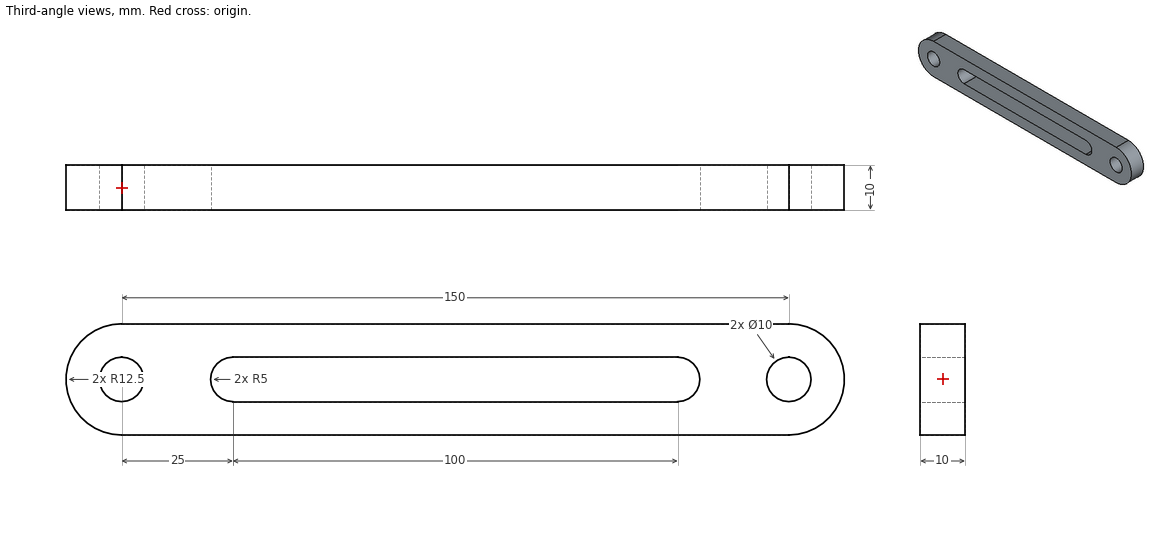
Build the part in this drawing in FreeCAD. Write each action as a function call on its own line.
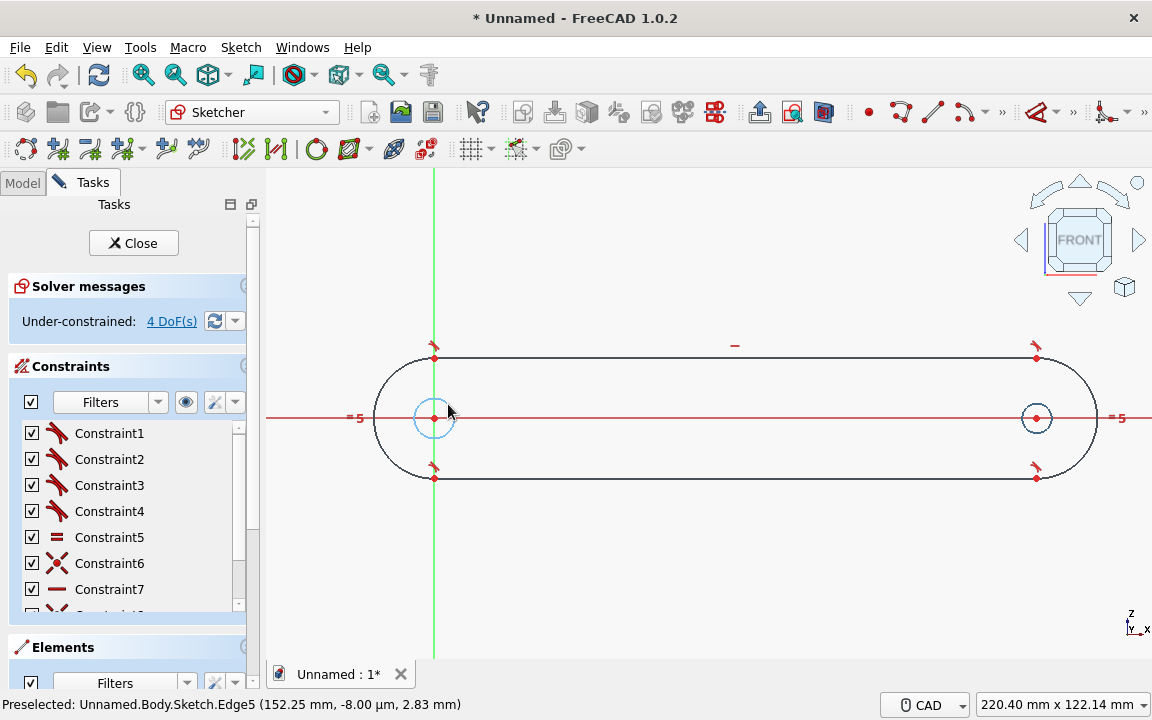
click(448, 404)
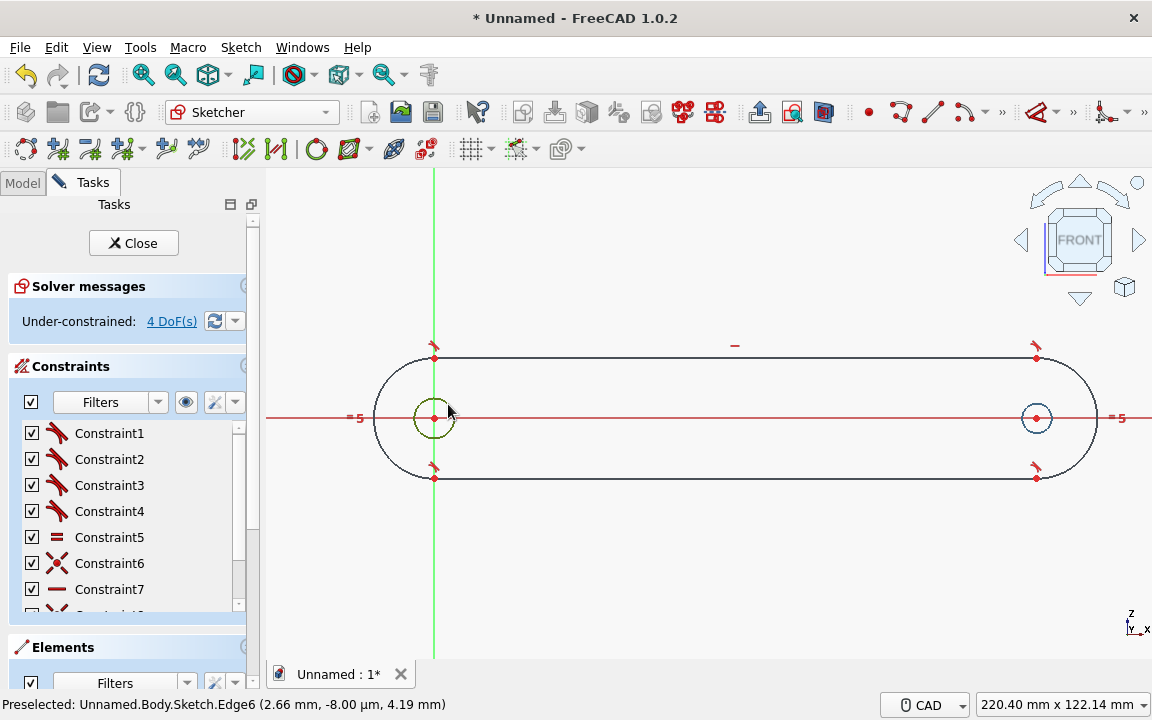
key(e)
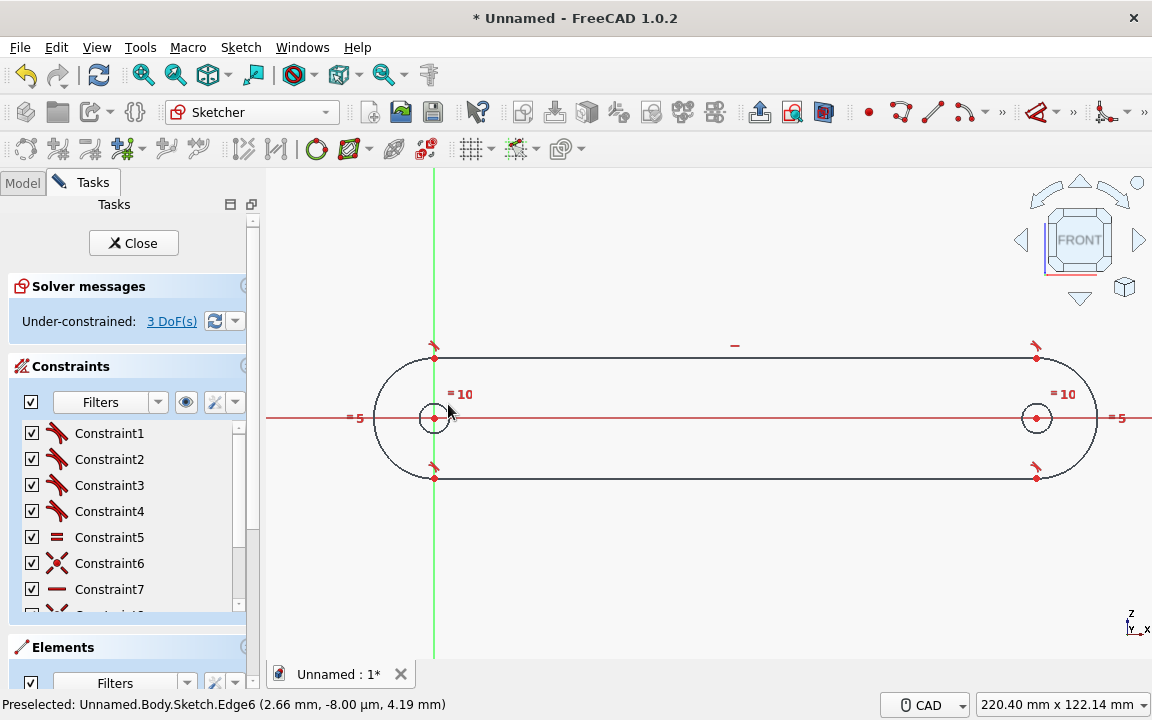
click(1036, 112)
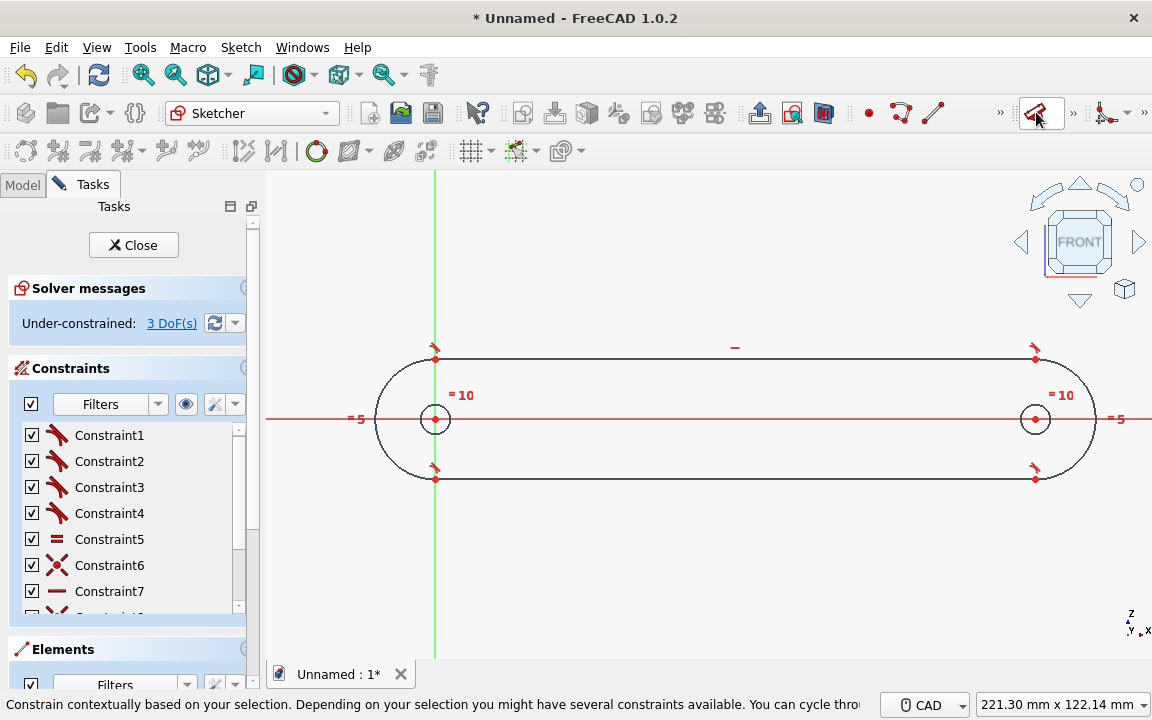
click(387, 384)
click(361, 365)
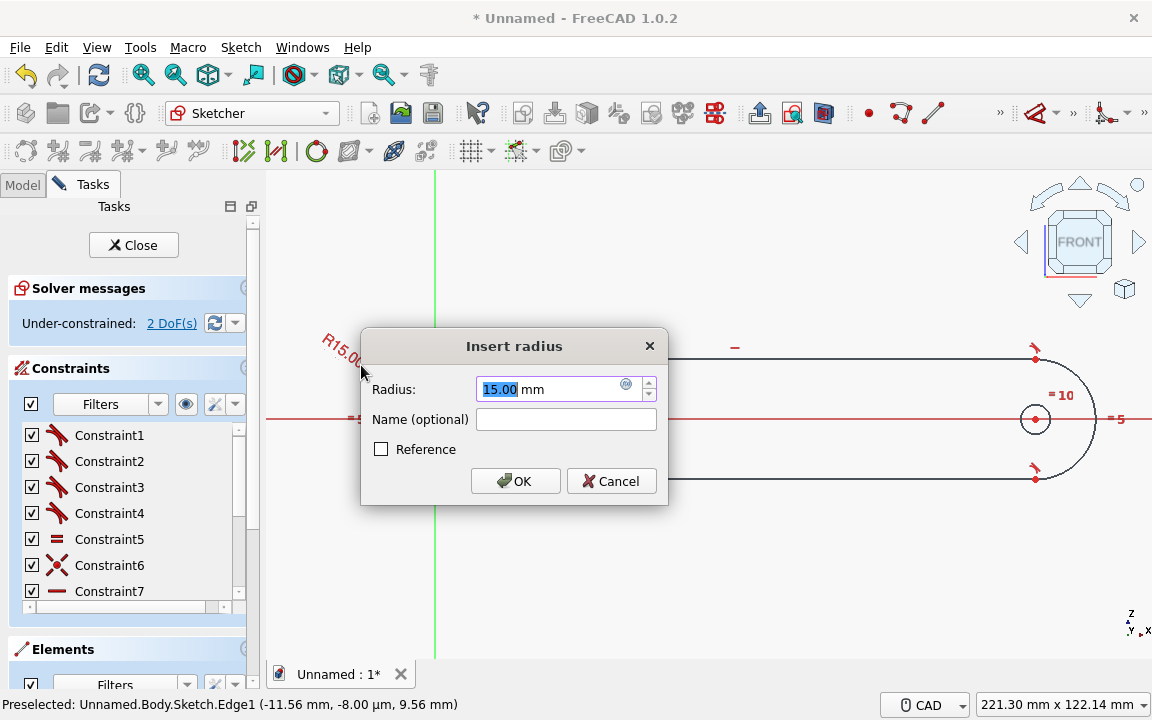
text(12.5)
key(Return)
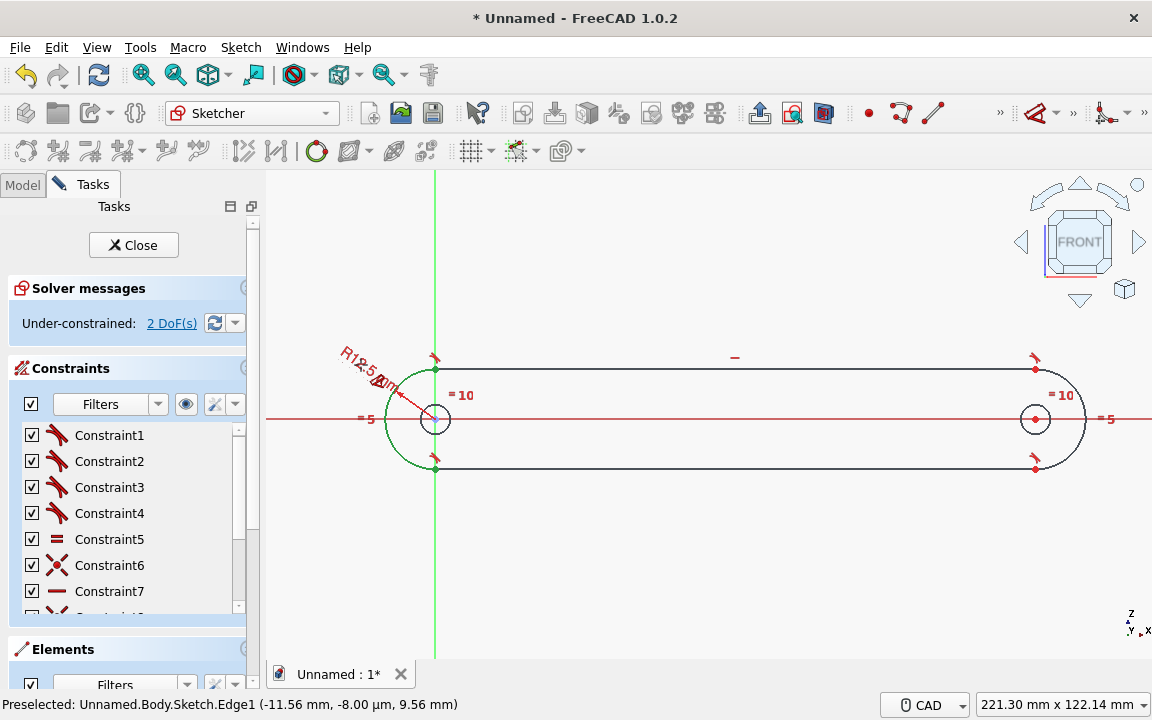
scroll(447, 405, down, 2)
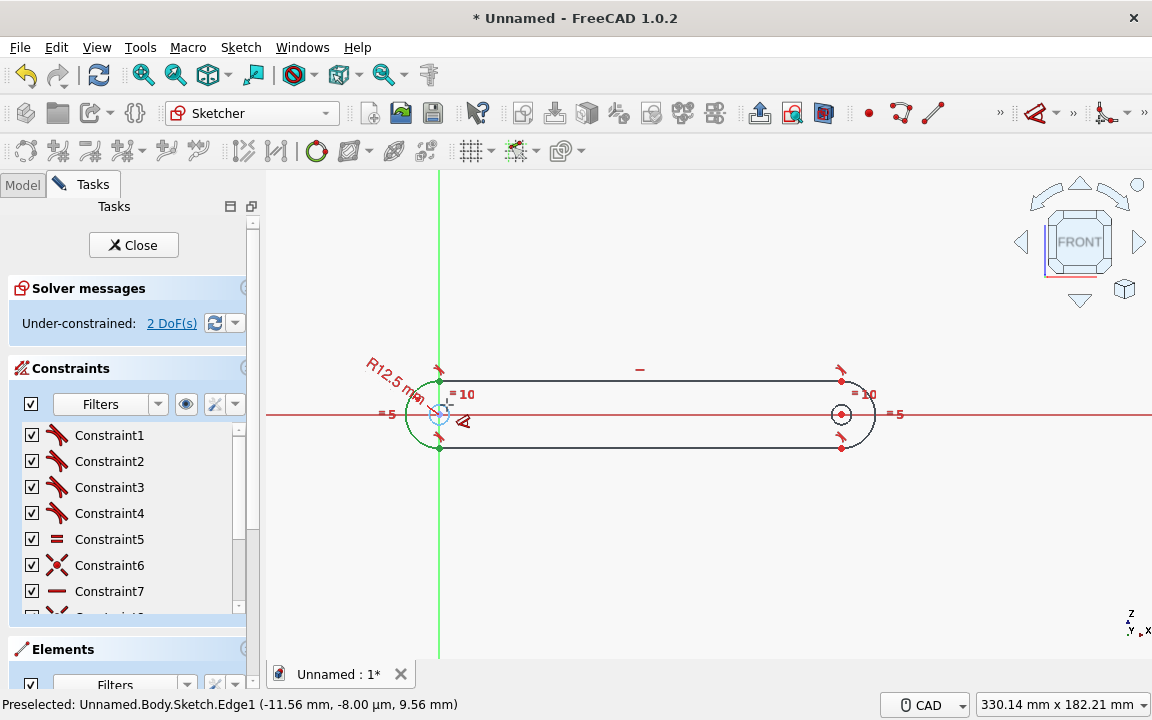
scroll(849, 408, up, 4)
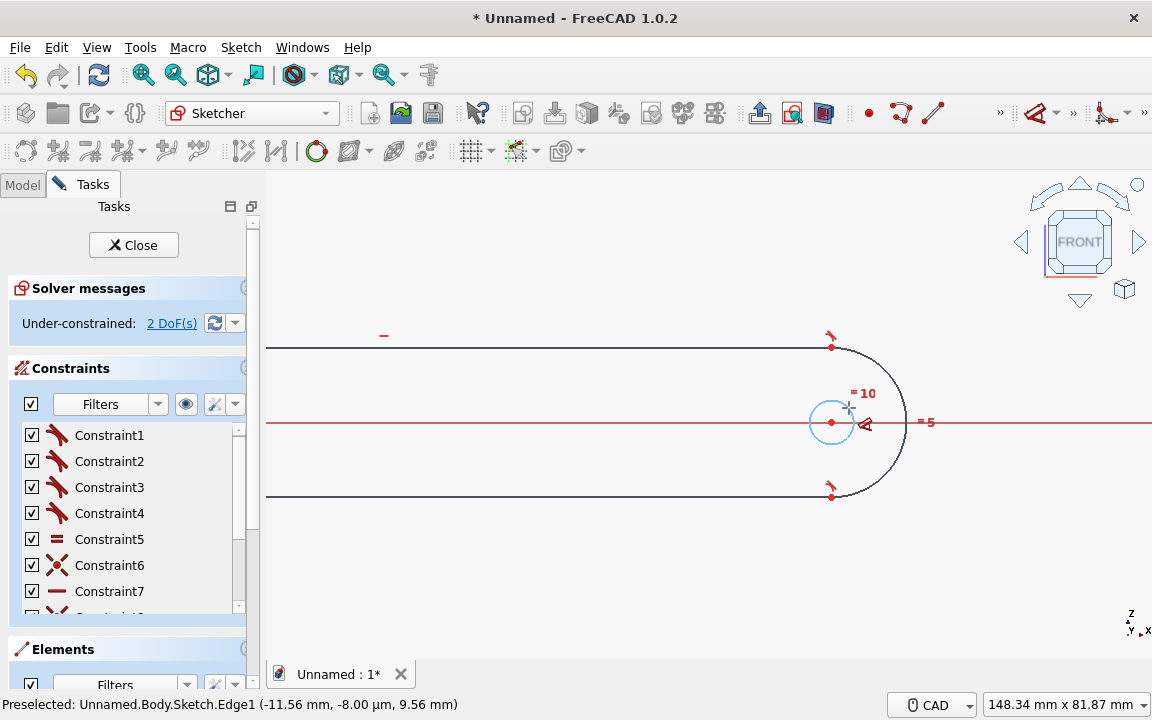
click(847, 407)
click(869, 384)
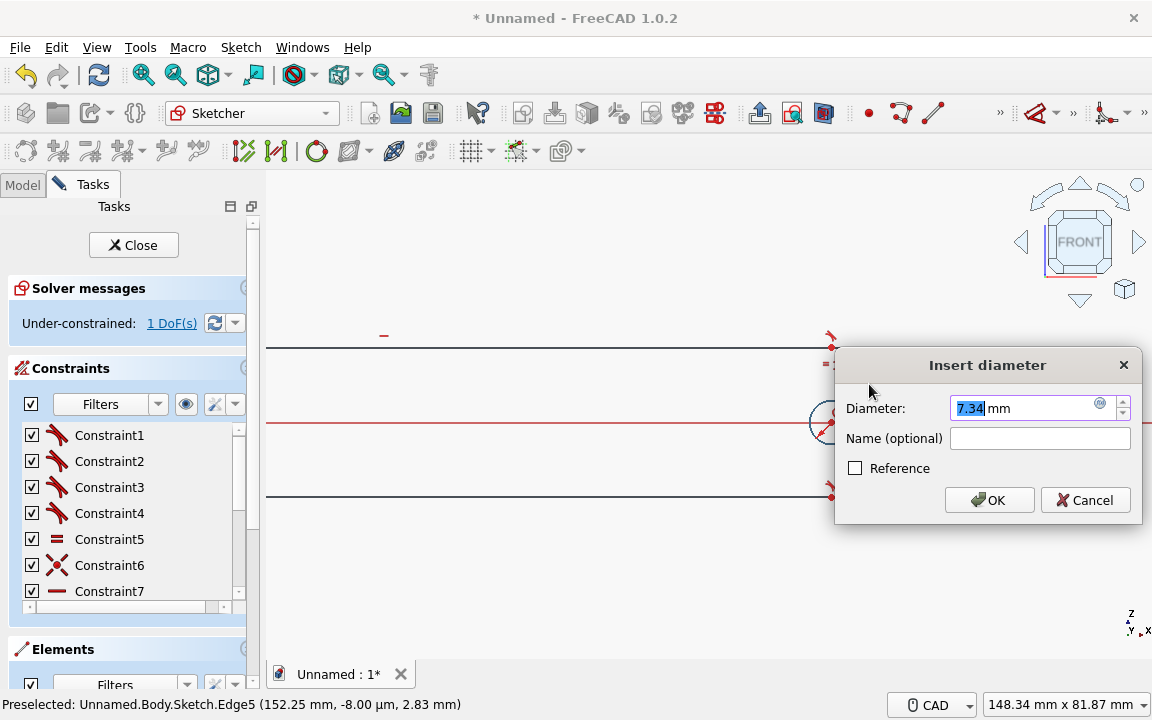
text(10)
key(Return)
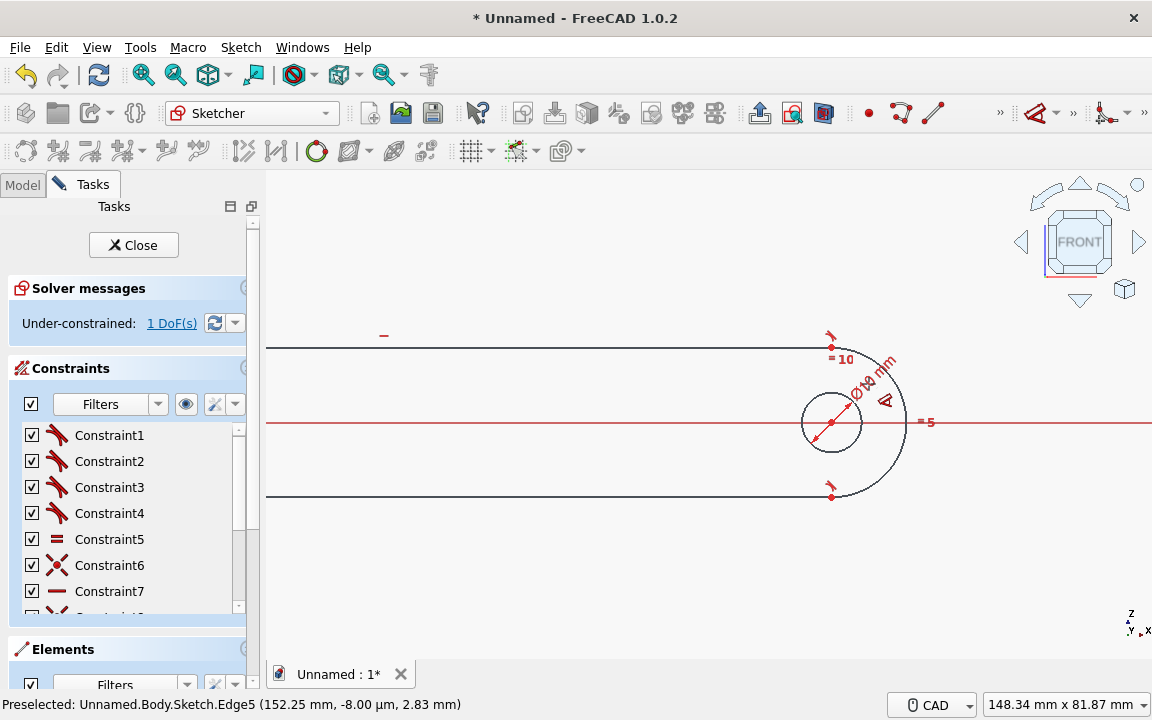
click(563, 348)
click(563, 314)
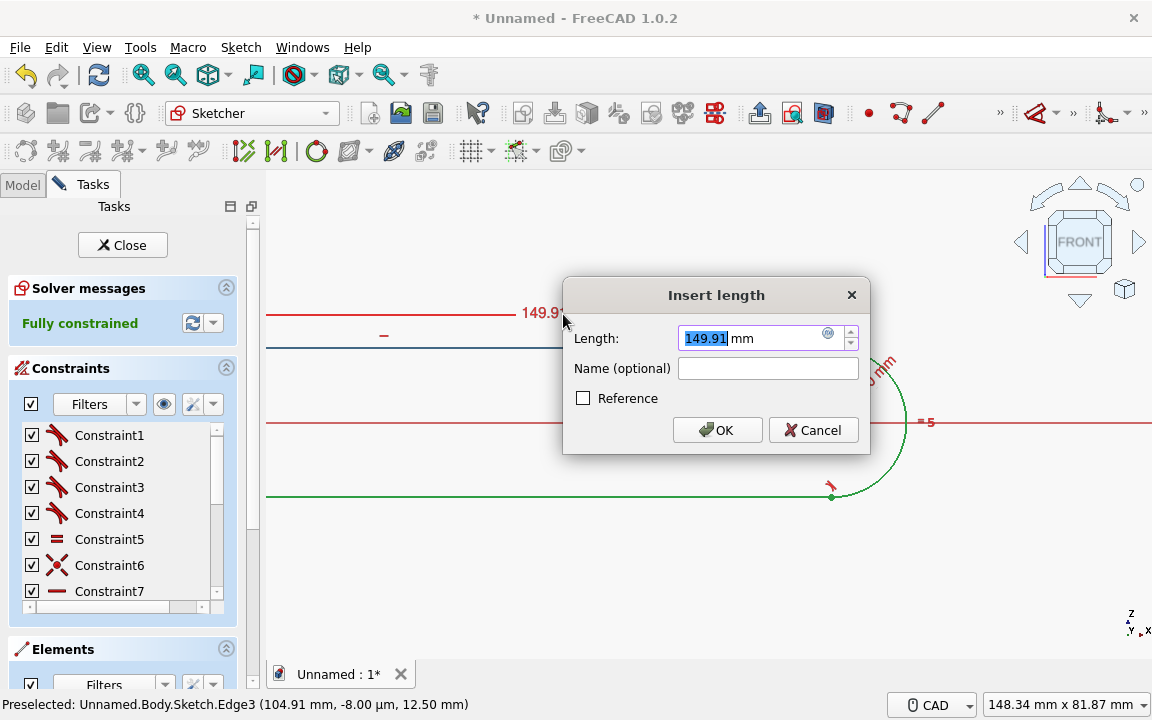
text(150)
key(Return)
key(Escape)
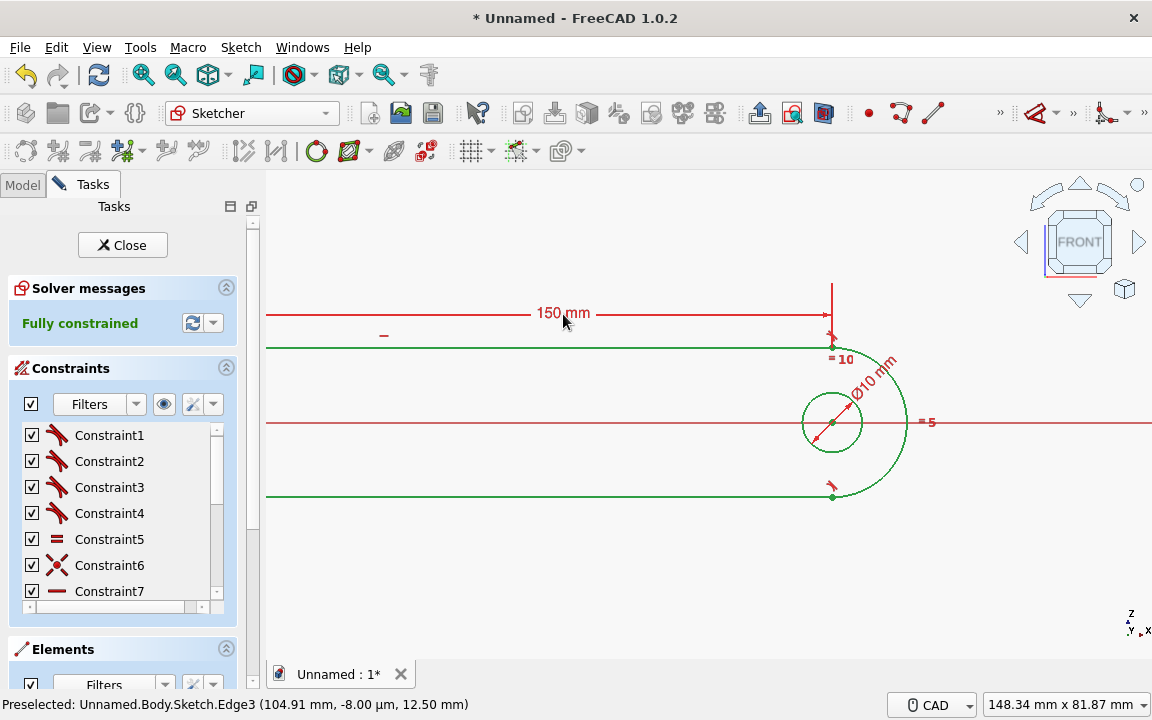
click(123, 245)